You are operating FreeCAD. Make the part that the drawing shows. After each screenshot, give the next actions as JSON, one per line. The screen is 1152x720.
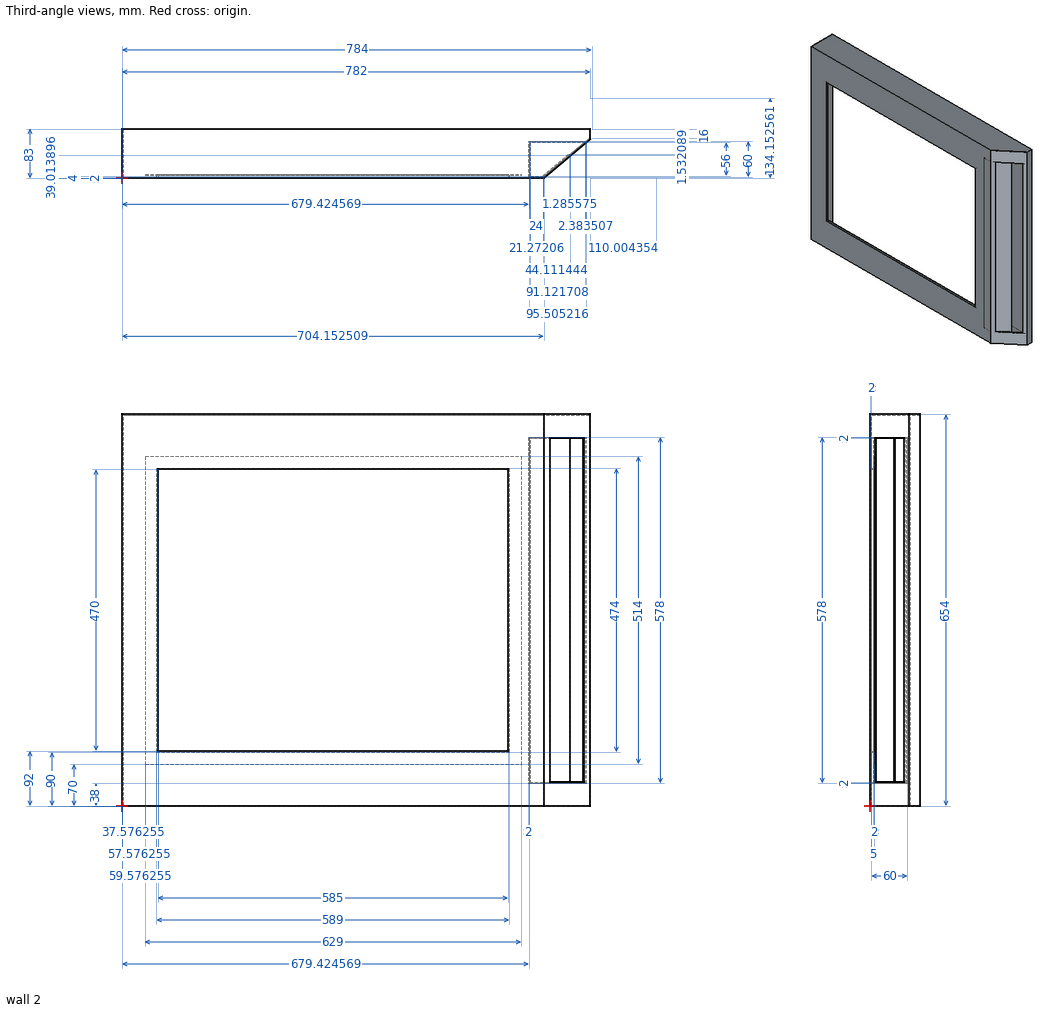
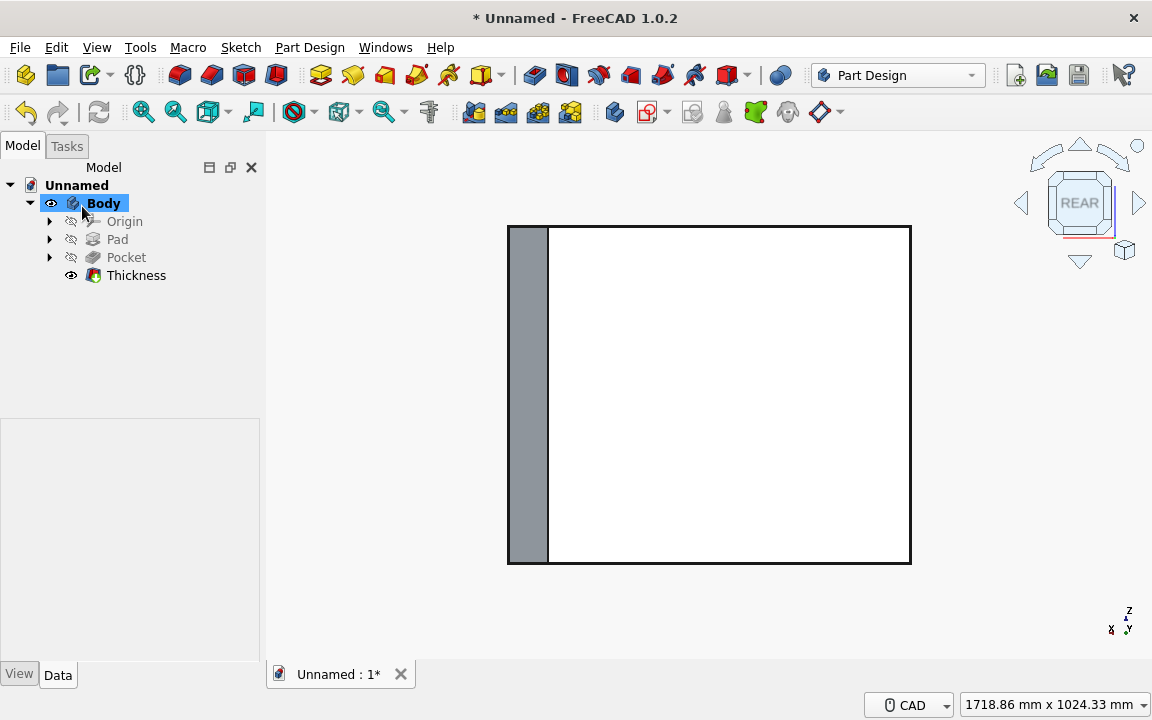
{"action": "key", "text": "0"}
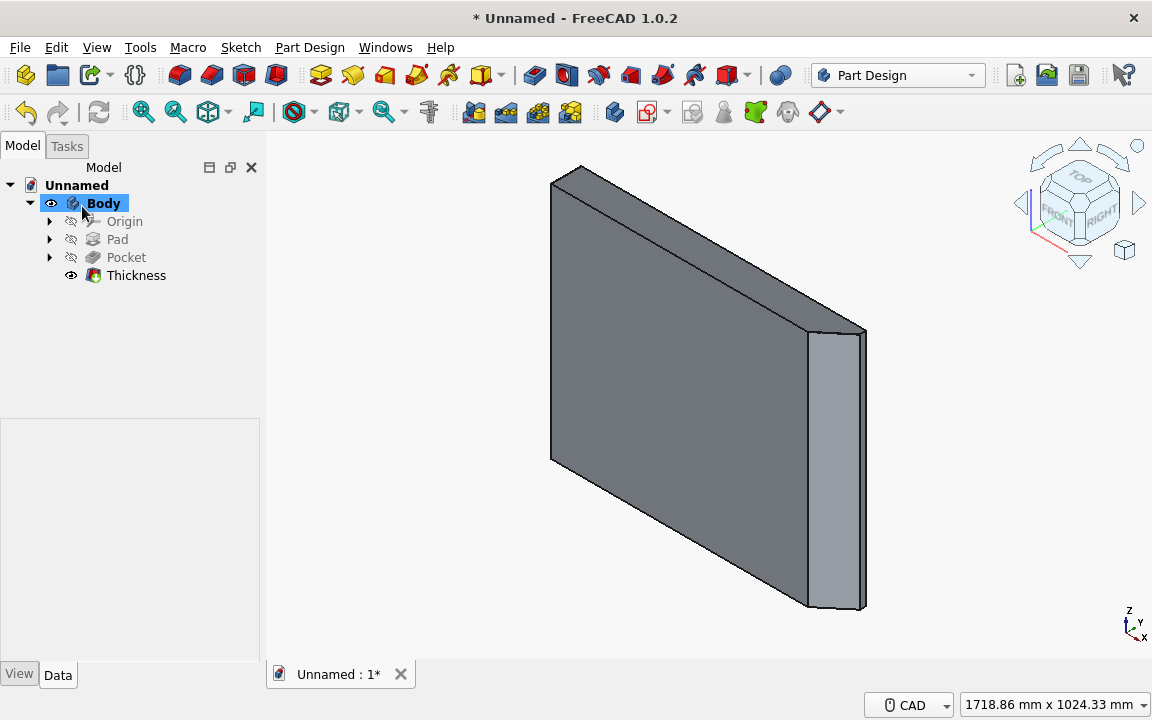
{"action": "left_click", "coordinate": [834, 391]}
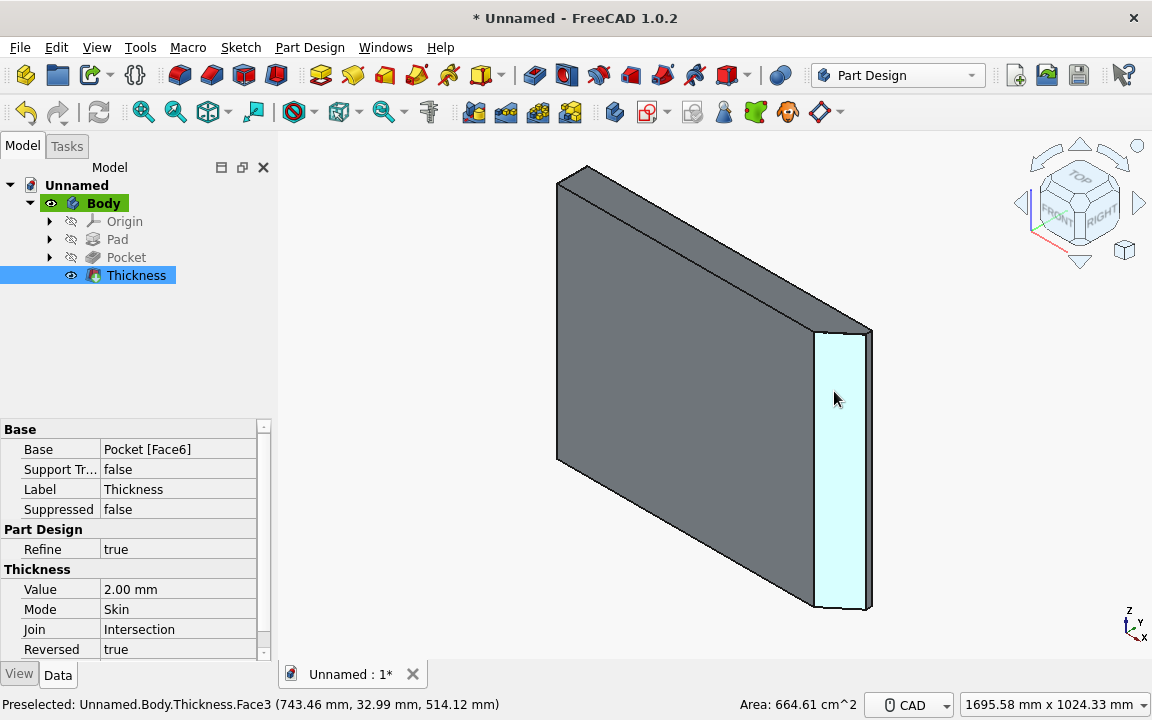
{"action": "left_click", "coordinate": [648, 112]}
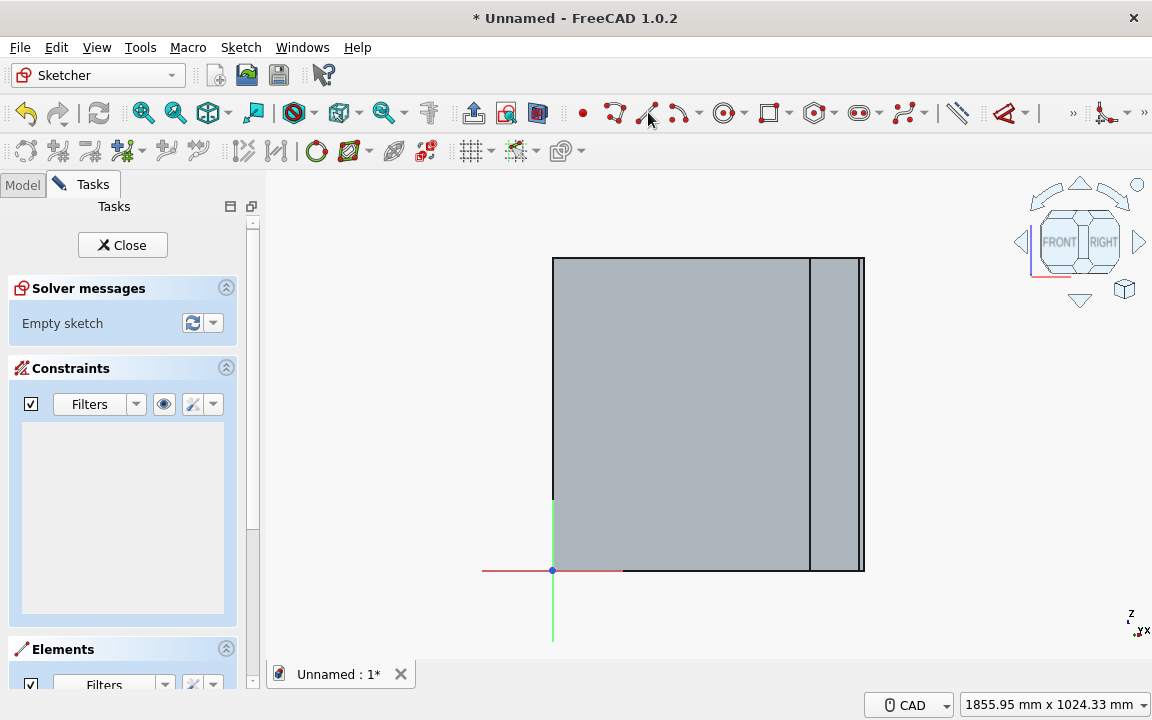
{"action": "key", "text": "q s"}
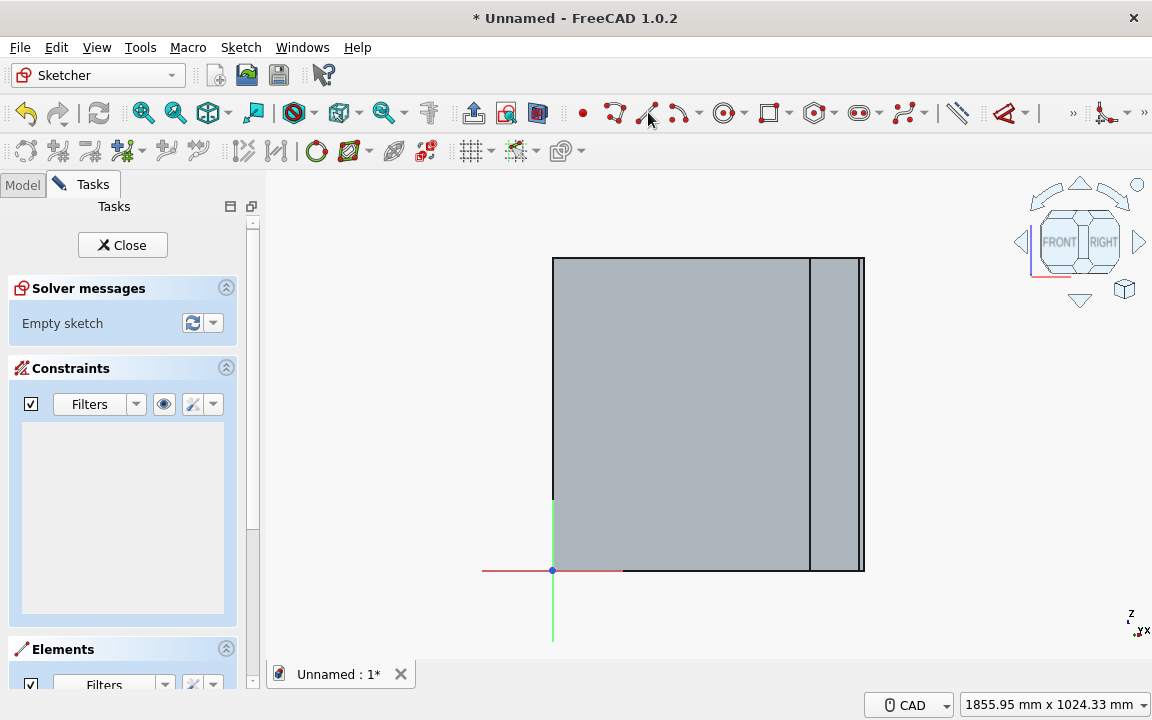
{"action": "key", "text": "g r"}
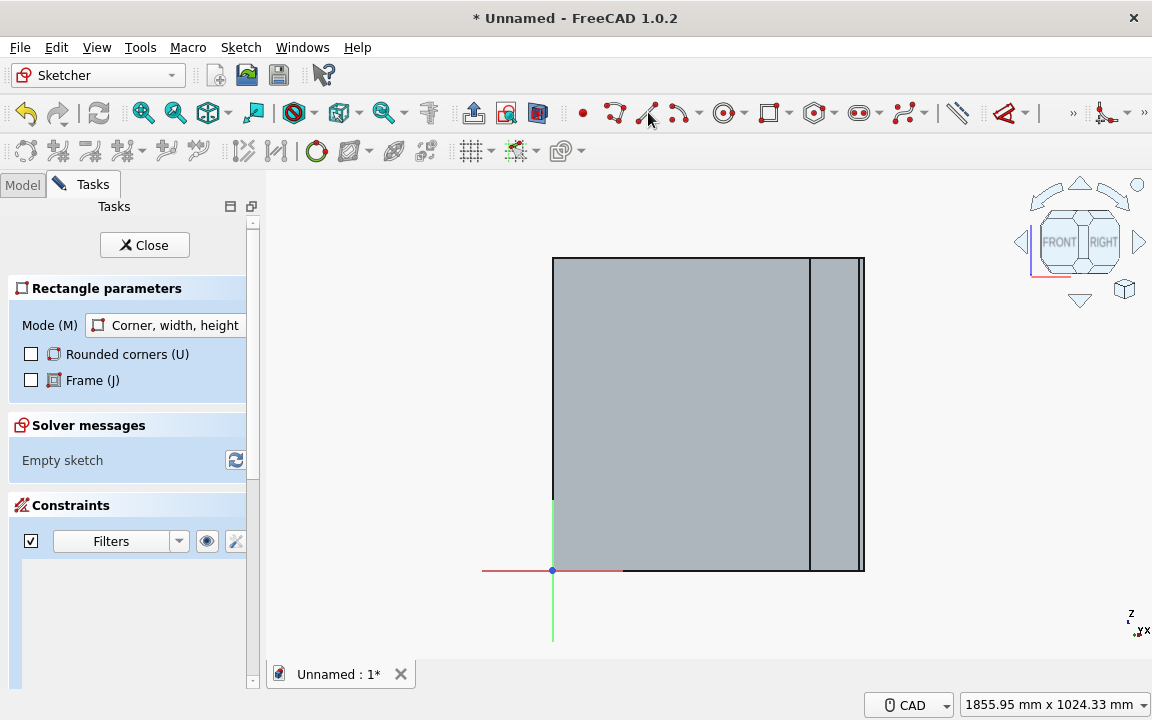
{"action": "left_click", "coordinate": [817, 277]}
{"action": "left_click", "coordinate": [853, 552]}
{"action": "key", "text": "Escape"}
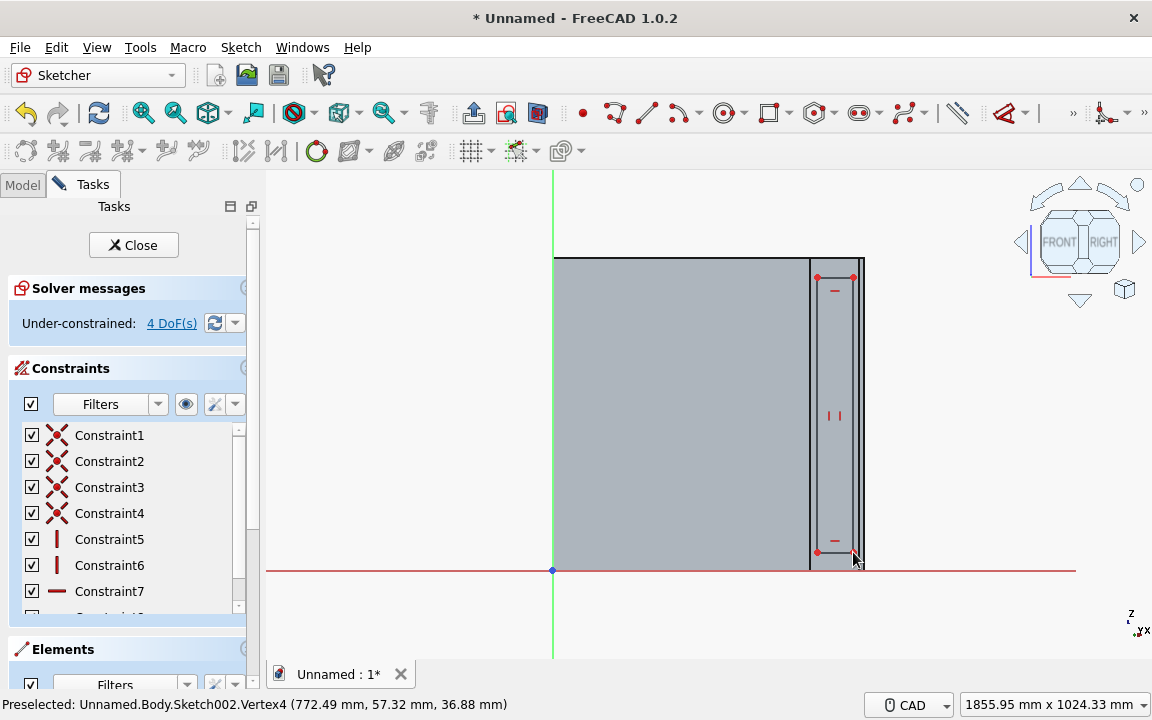
{"action": "key", "text": "d"}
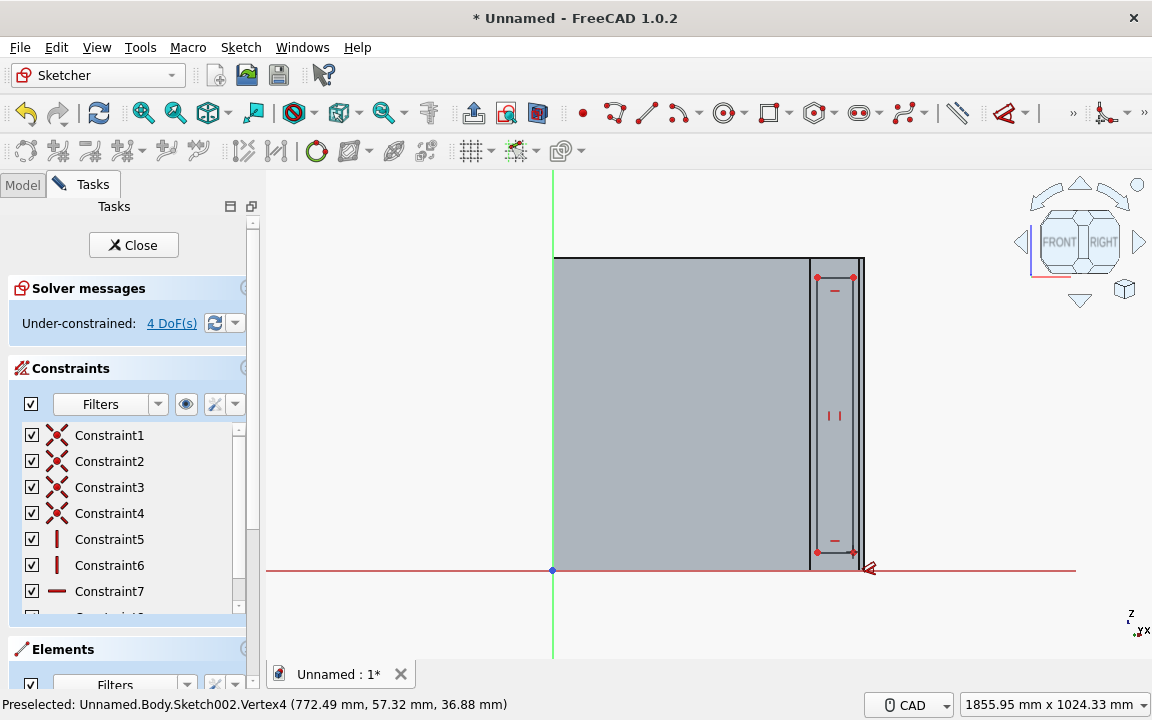
{"action": "scroll", "coordinate": [828, 553], "scroll_direction": "up", "scroll_amount": 2}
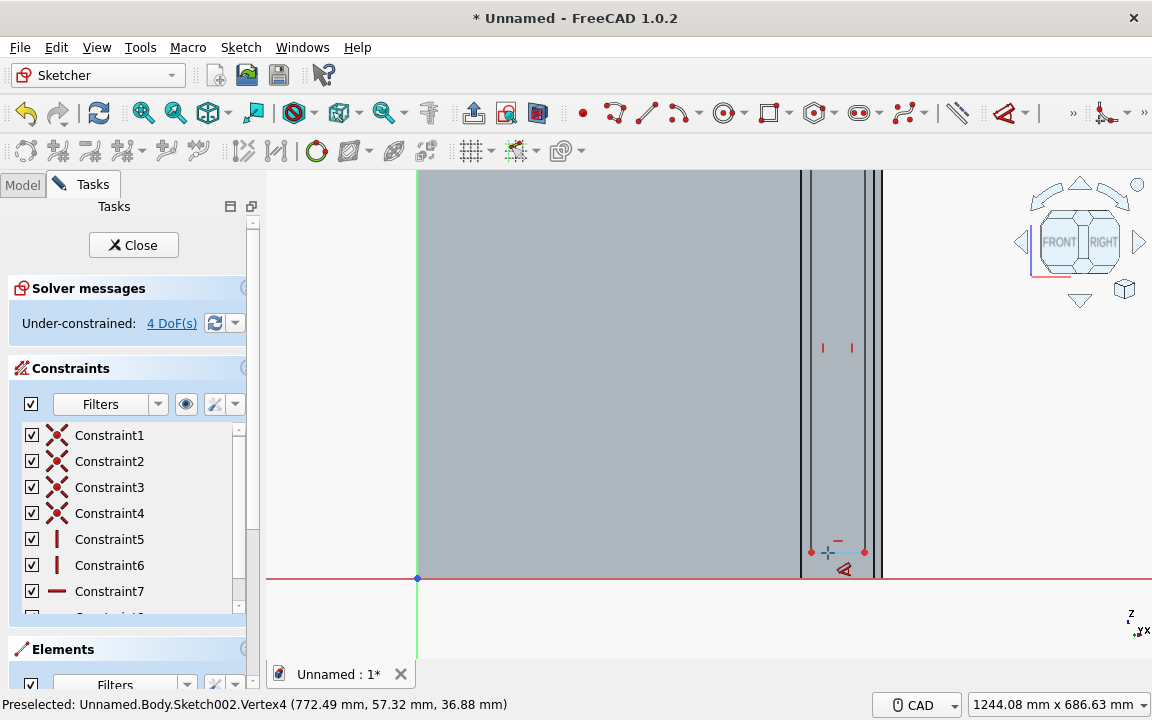
{"action": "left_click", "coordinate": [827, 553]}
{"action": "left_click", "coordinate": [838, 519]}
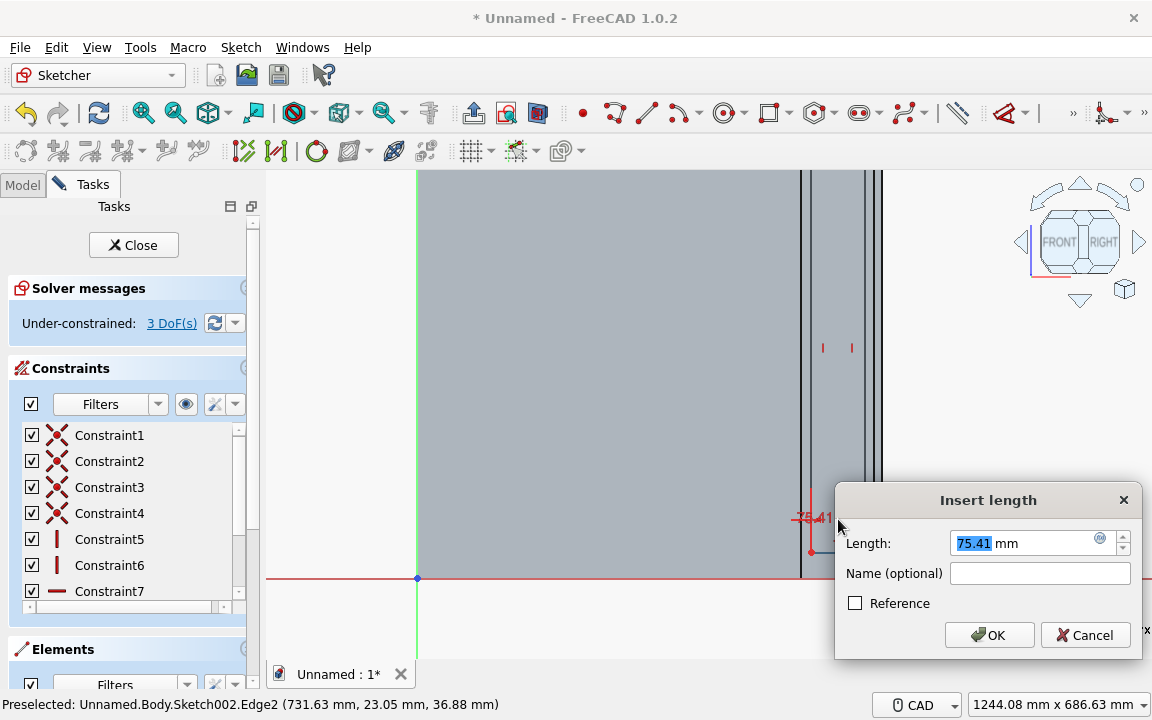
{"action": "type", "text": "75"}
{"action": "key", "text": "Return"}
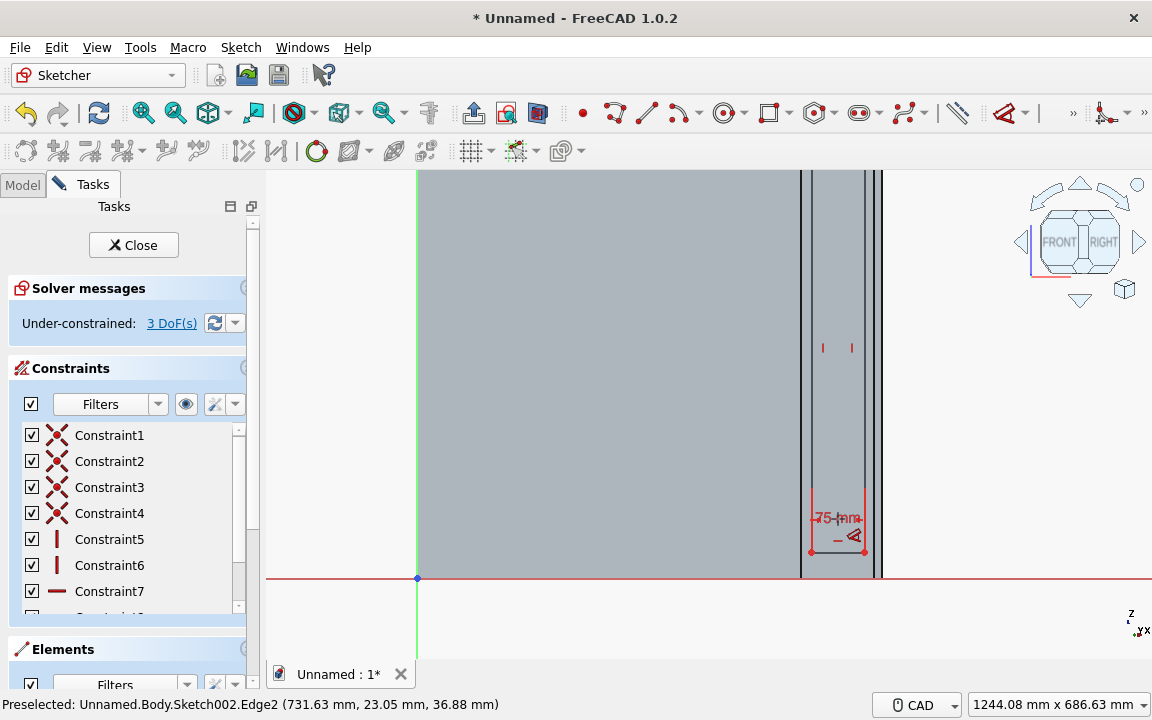
{"action": "left_click", "coordinate": [812, 265]}
{"action": "left_click", "coordinate": [846, 375]}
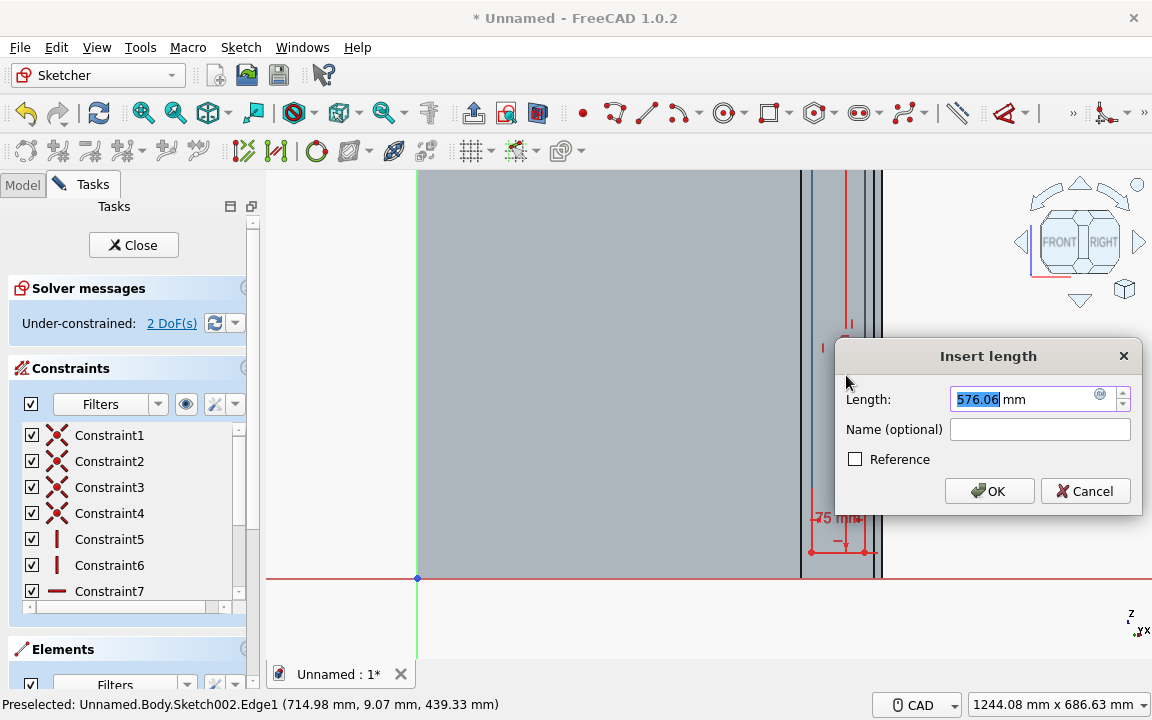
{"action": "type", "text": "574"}
{"action": "key", "text": "Return"}